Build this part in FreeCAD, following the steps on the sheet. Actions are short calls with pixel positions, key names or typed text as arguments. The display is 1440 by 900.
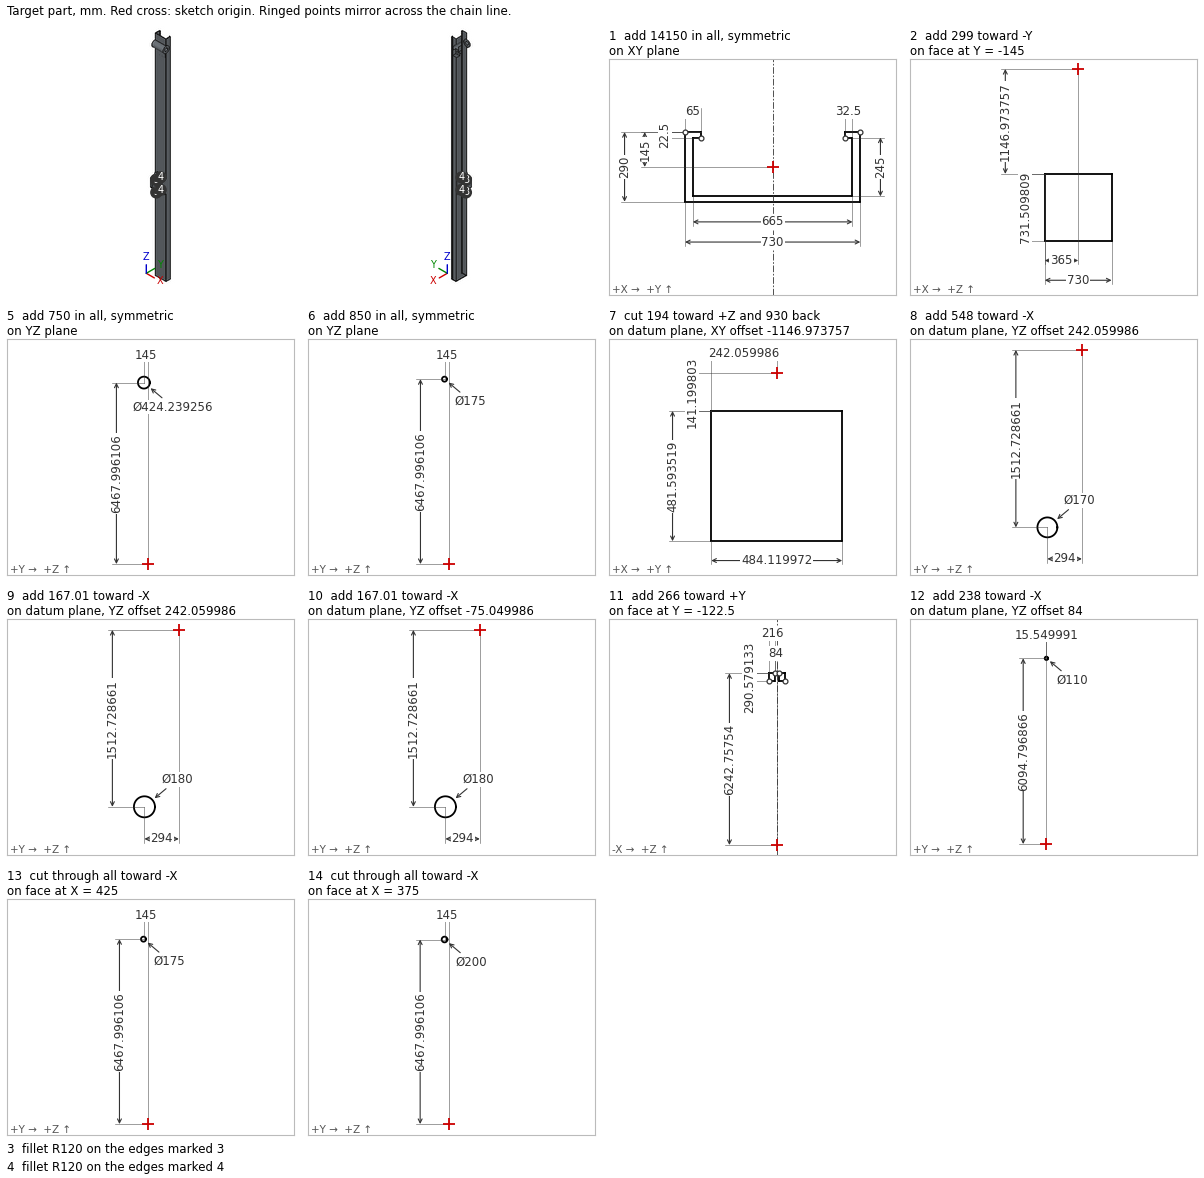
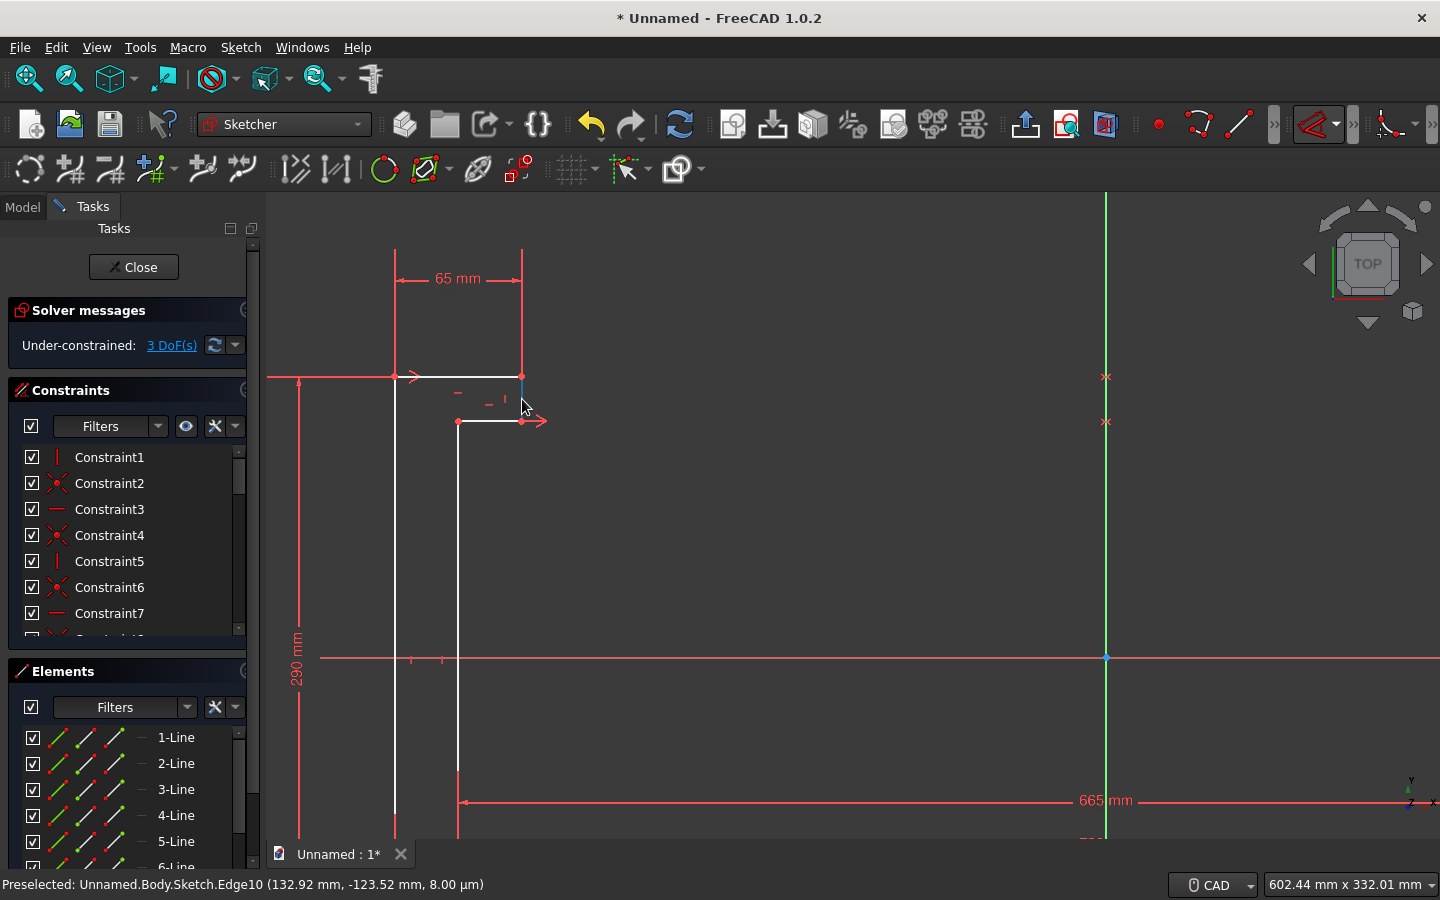
click(522, 399)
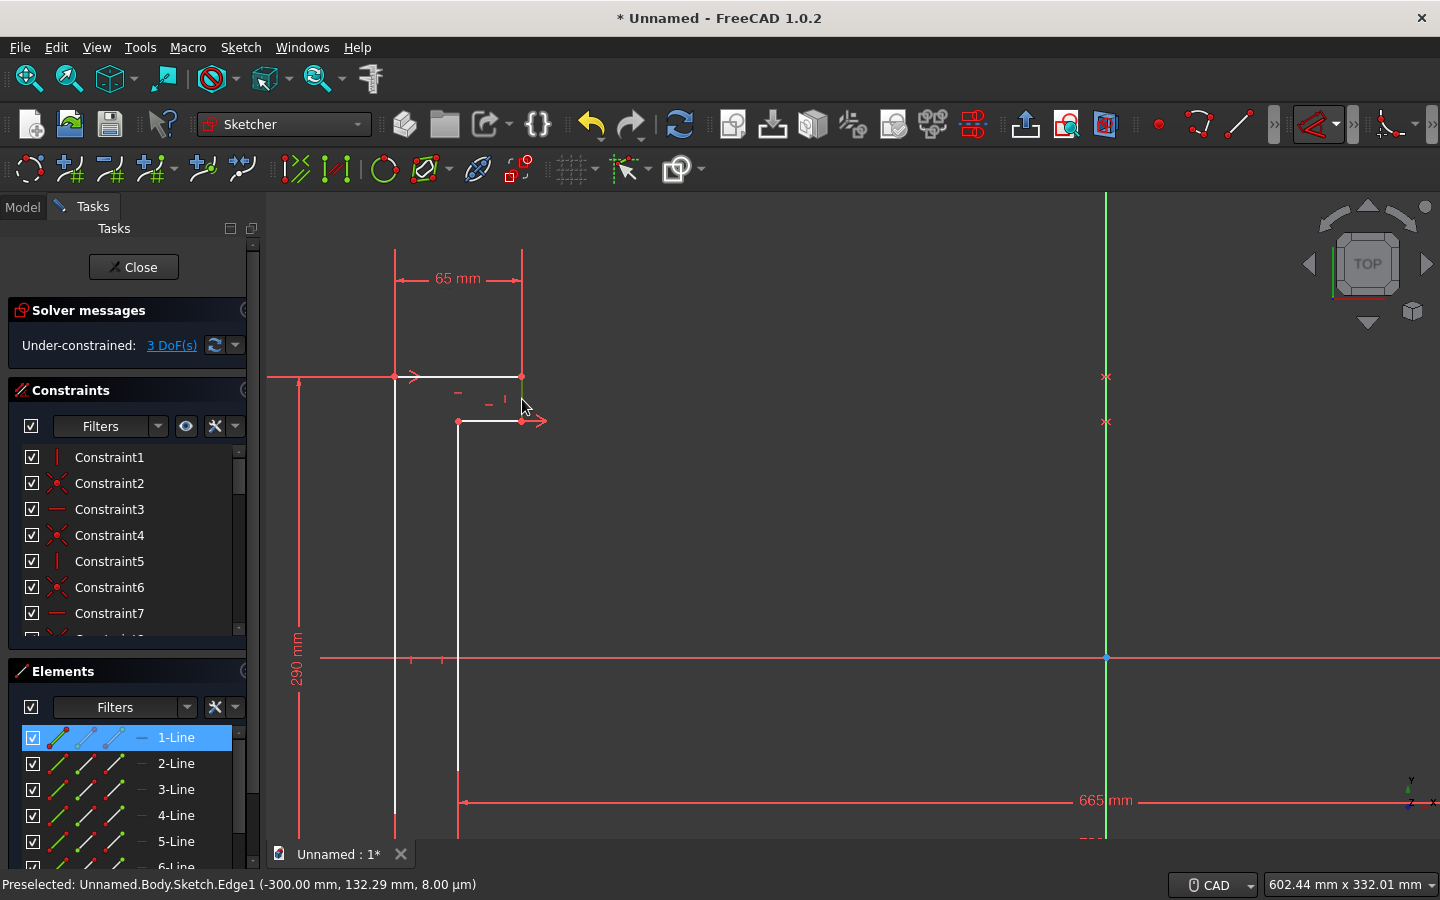
click(1338, 124)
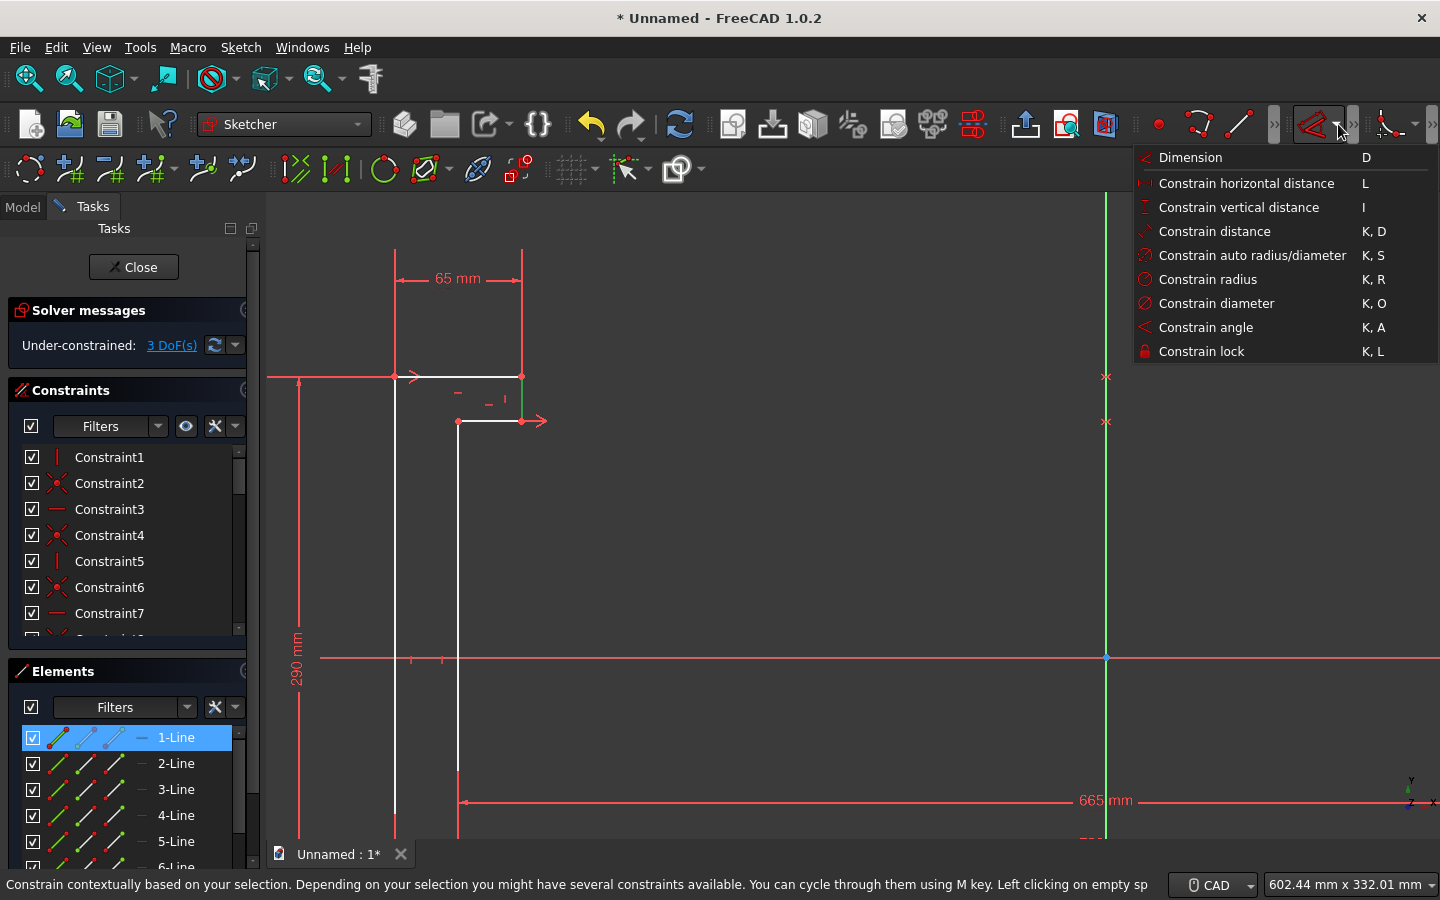
click(1286, 207)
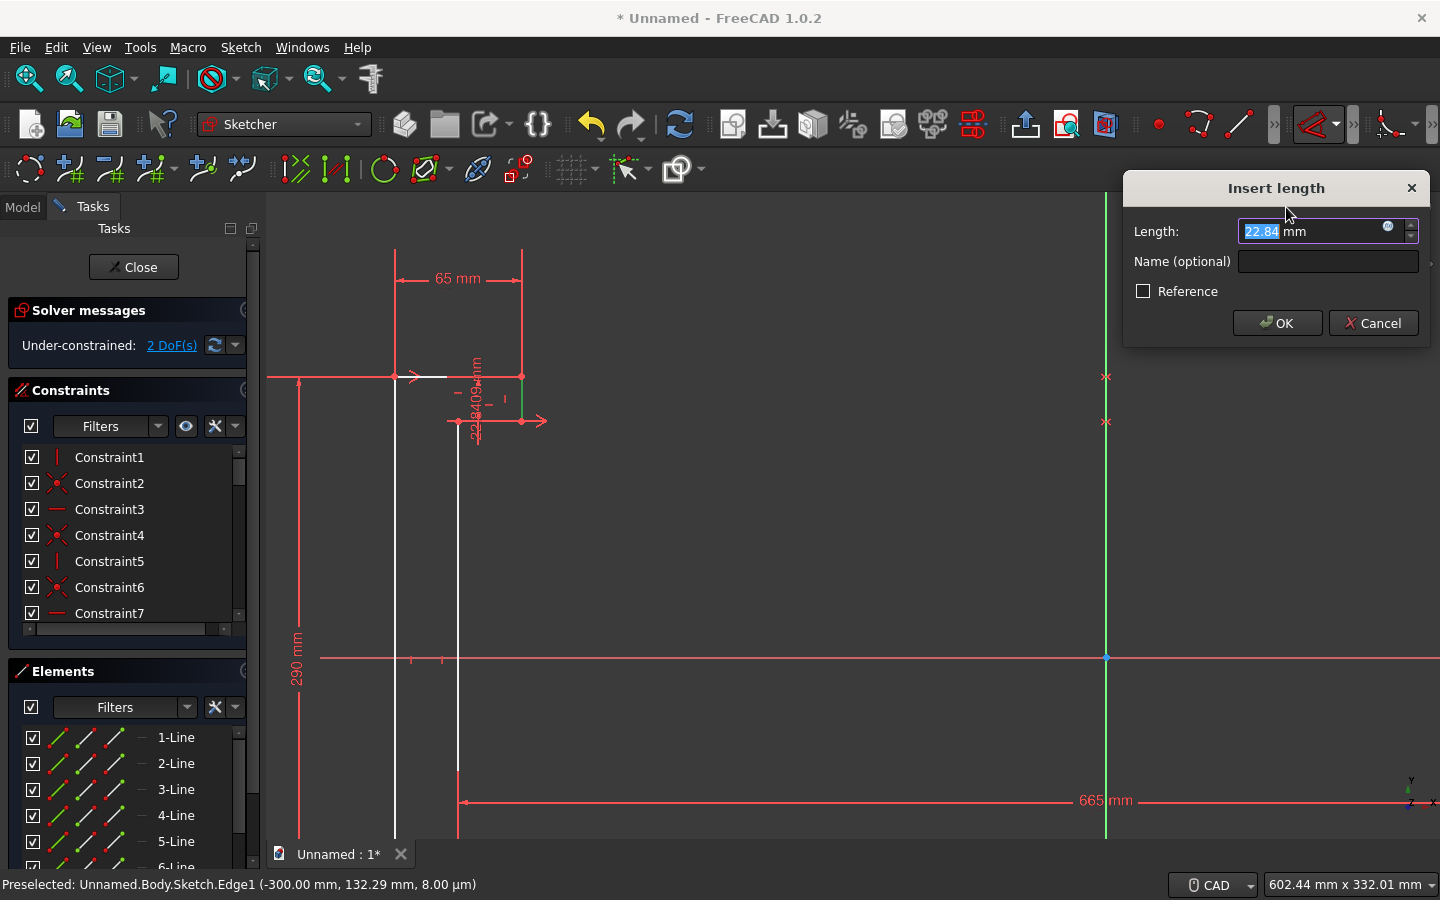
text(22.5)
key(Return)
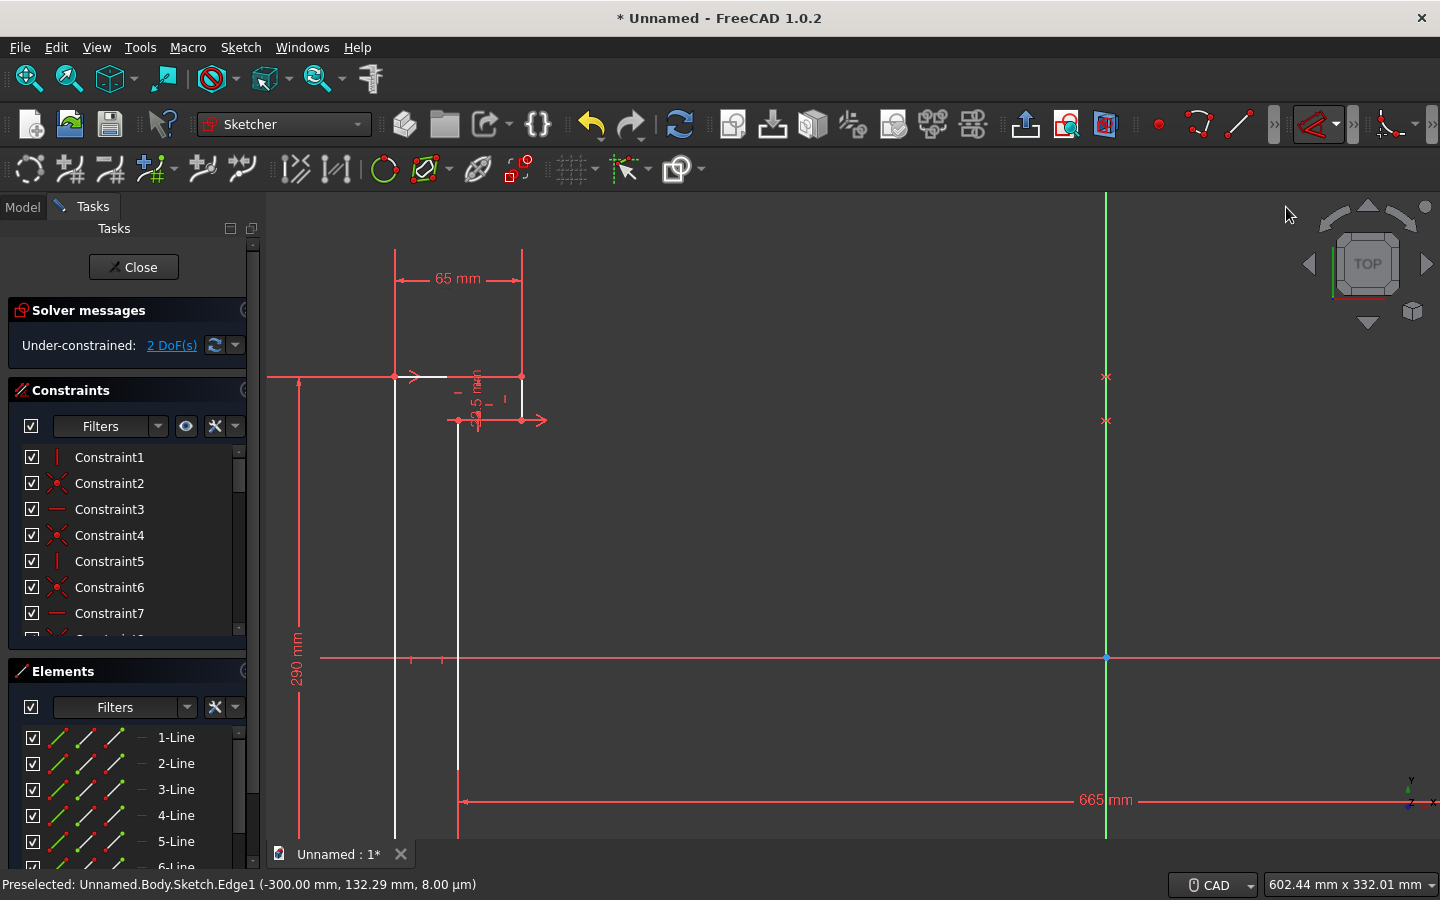
scroll(522, 399, down, 4)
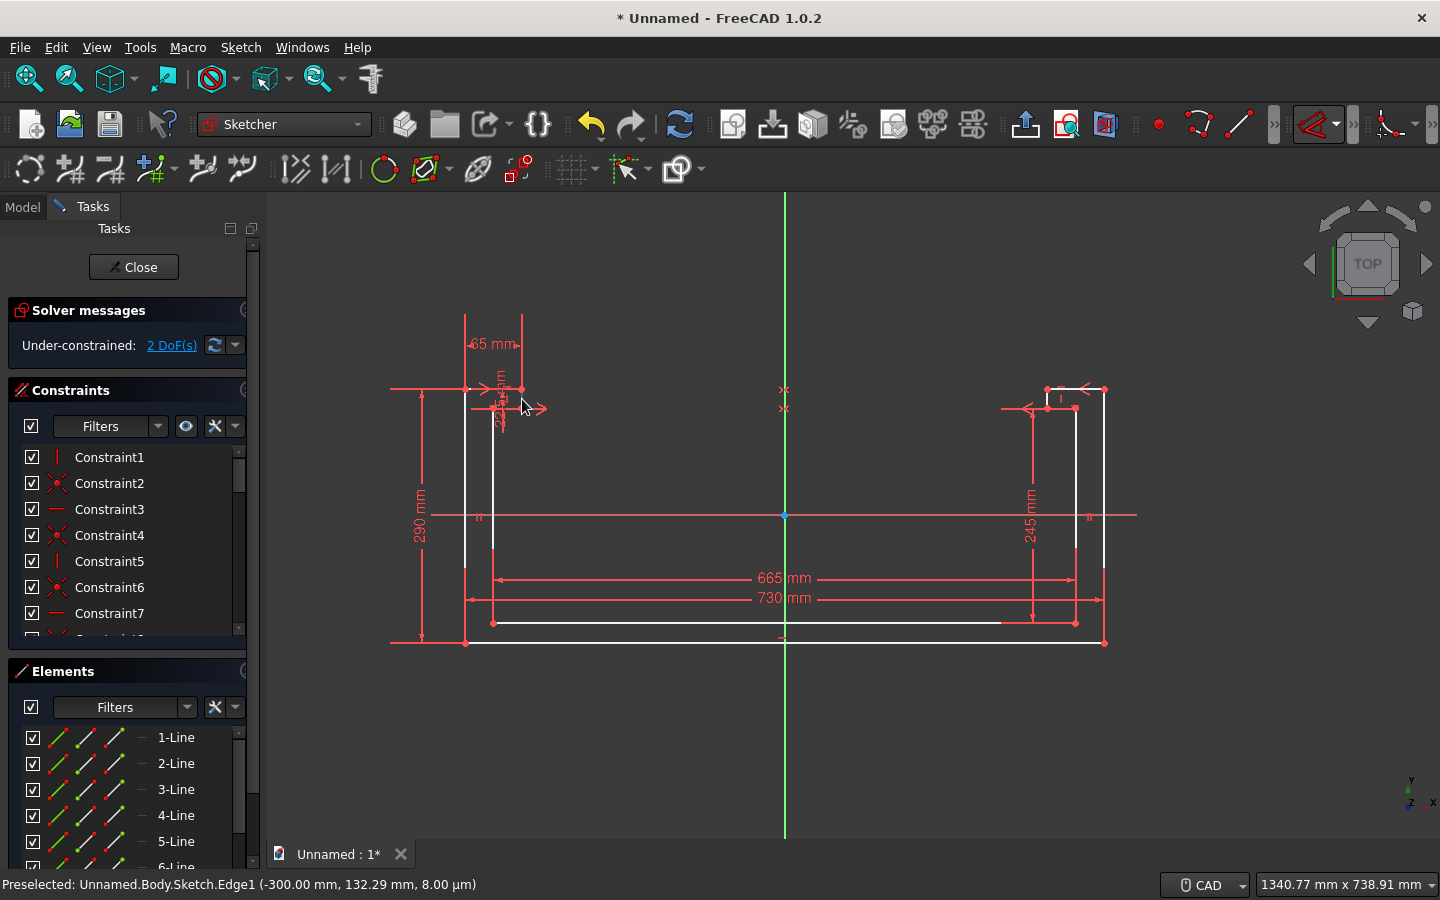
scroll(1056, 409, up, 3)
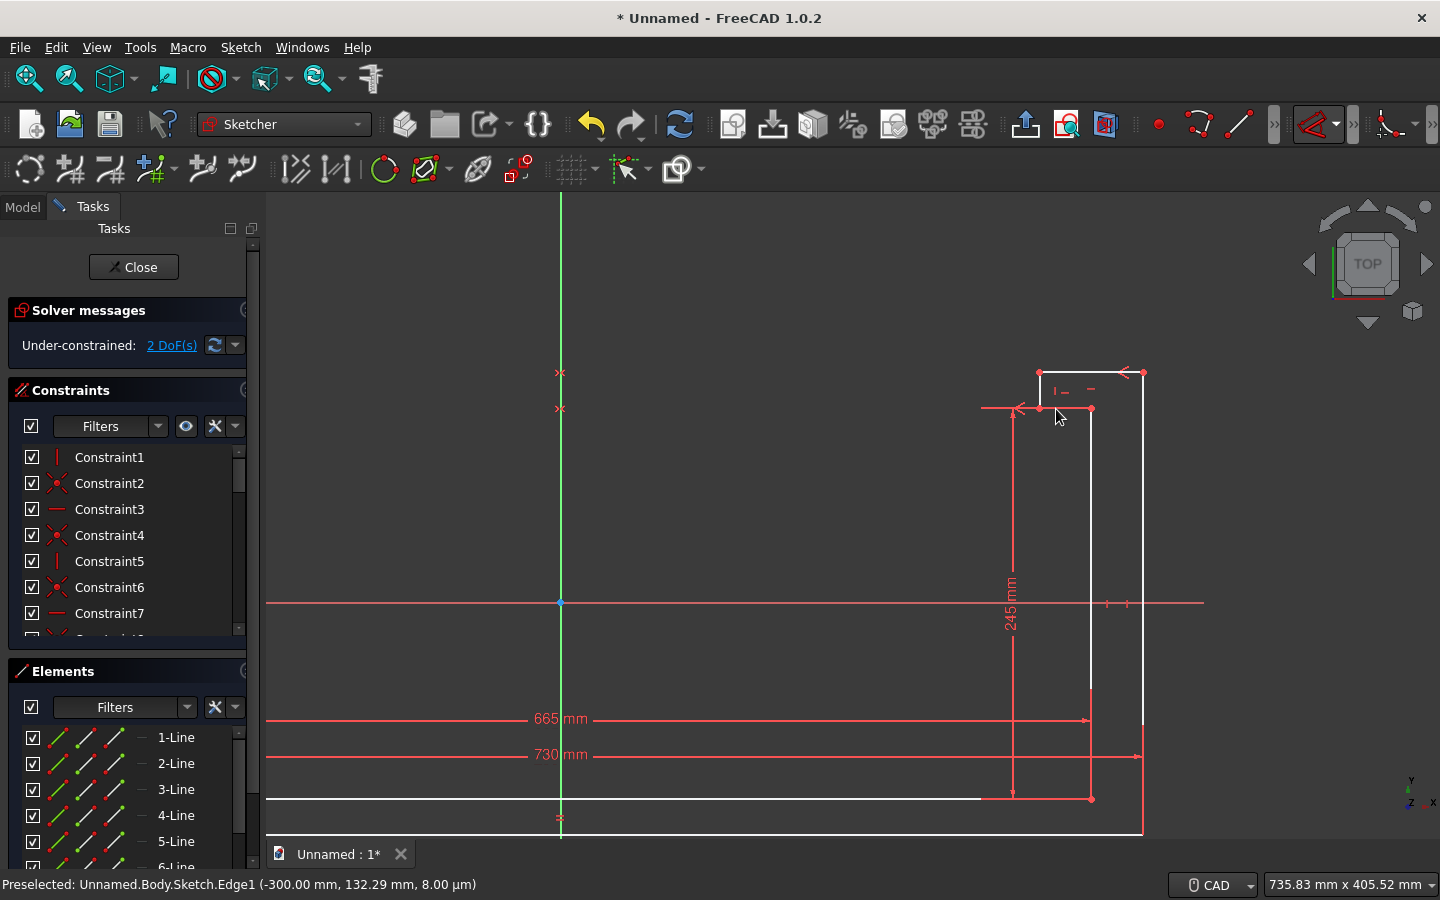
click(1055, 408)